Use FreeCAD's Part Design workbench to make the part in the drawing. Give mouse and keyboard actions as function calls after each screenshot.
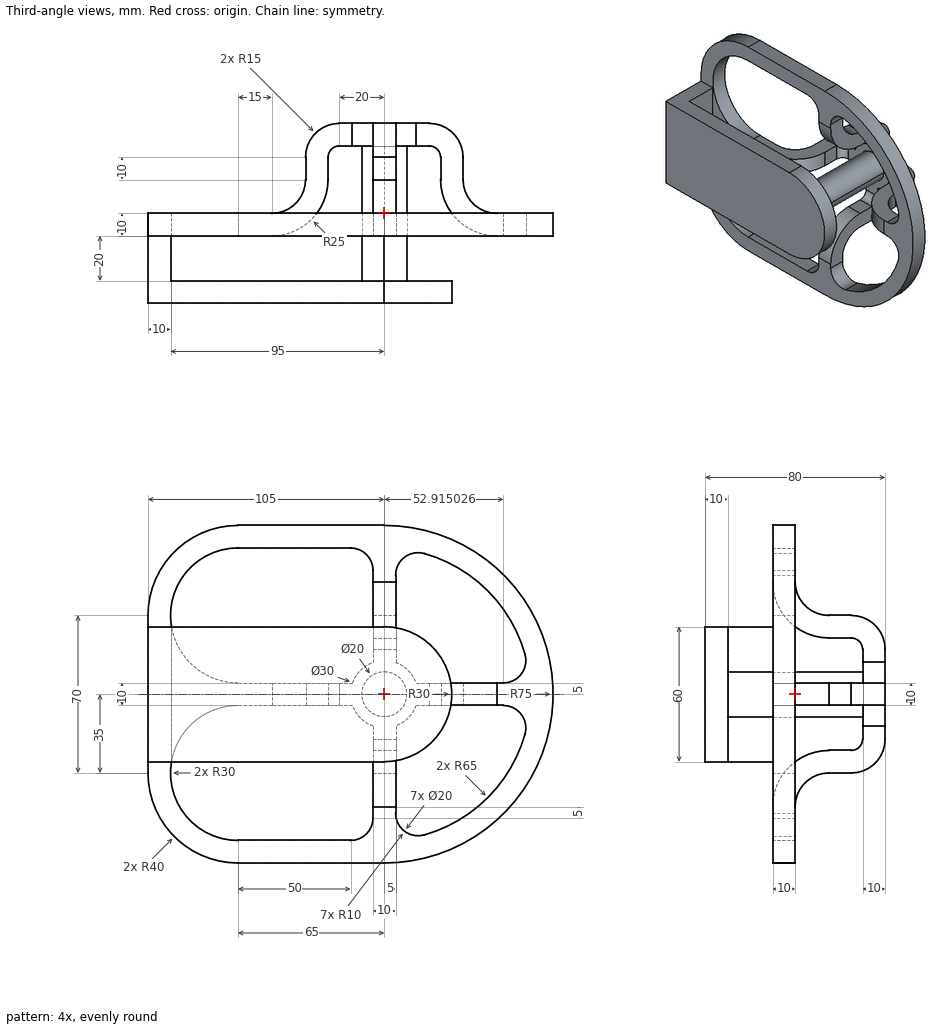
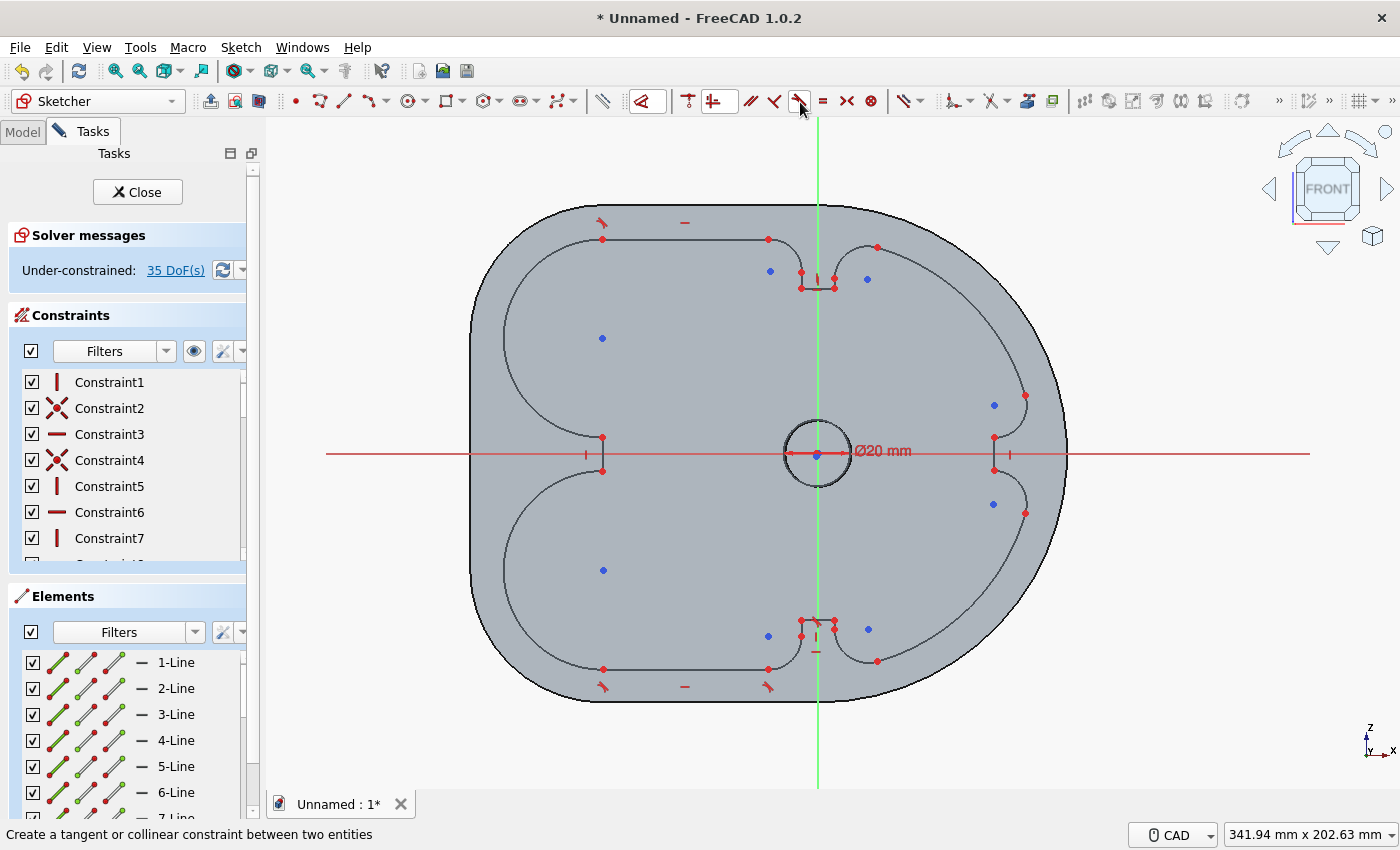
click(653, 240)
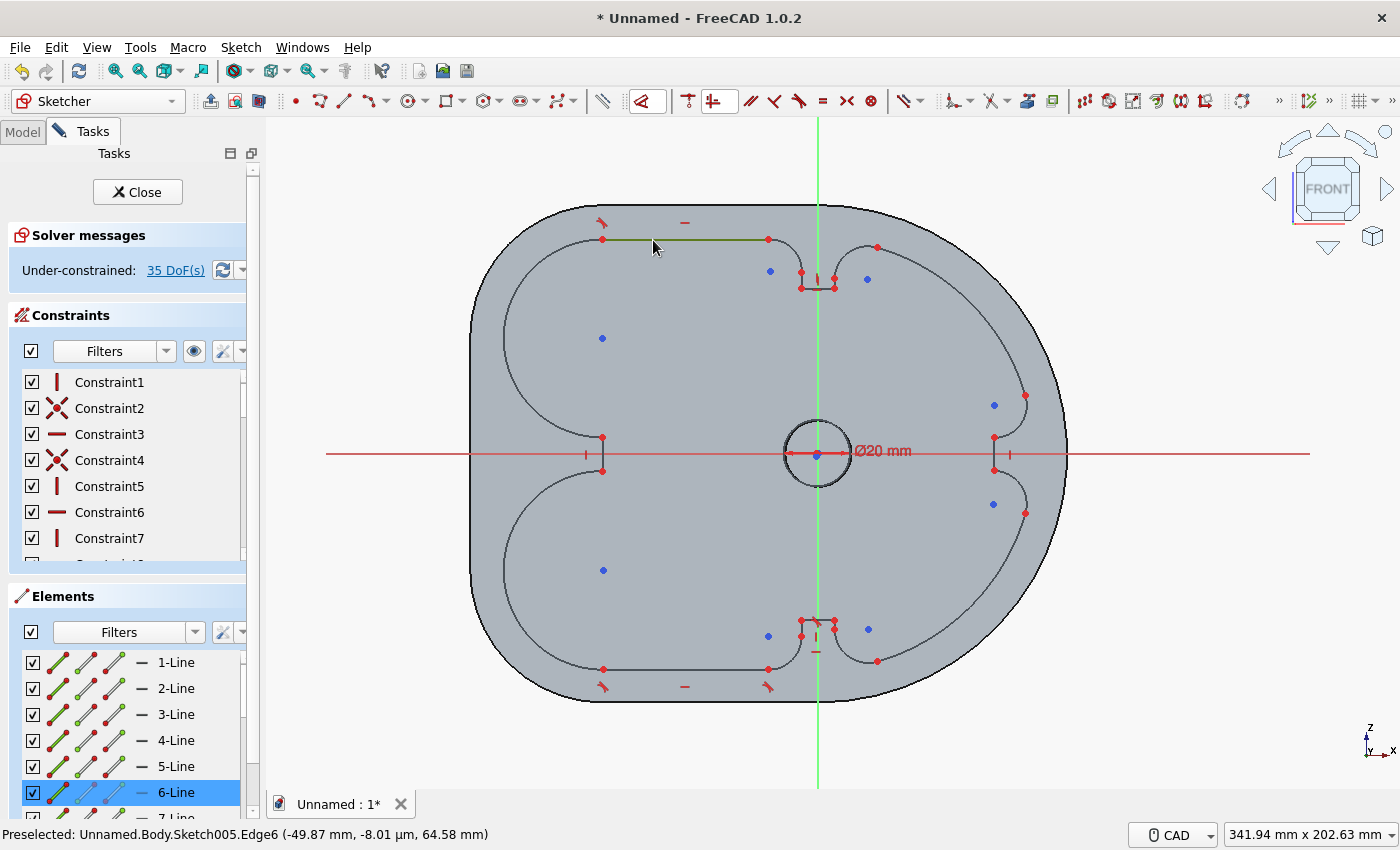
click(799, 257)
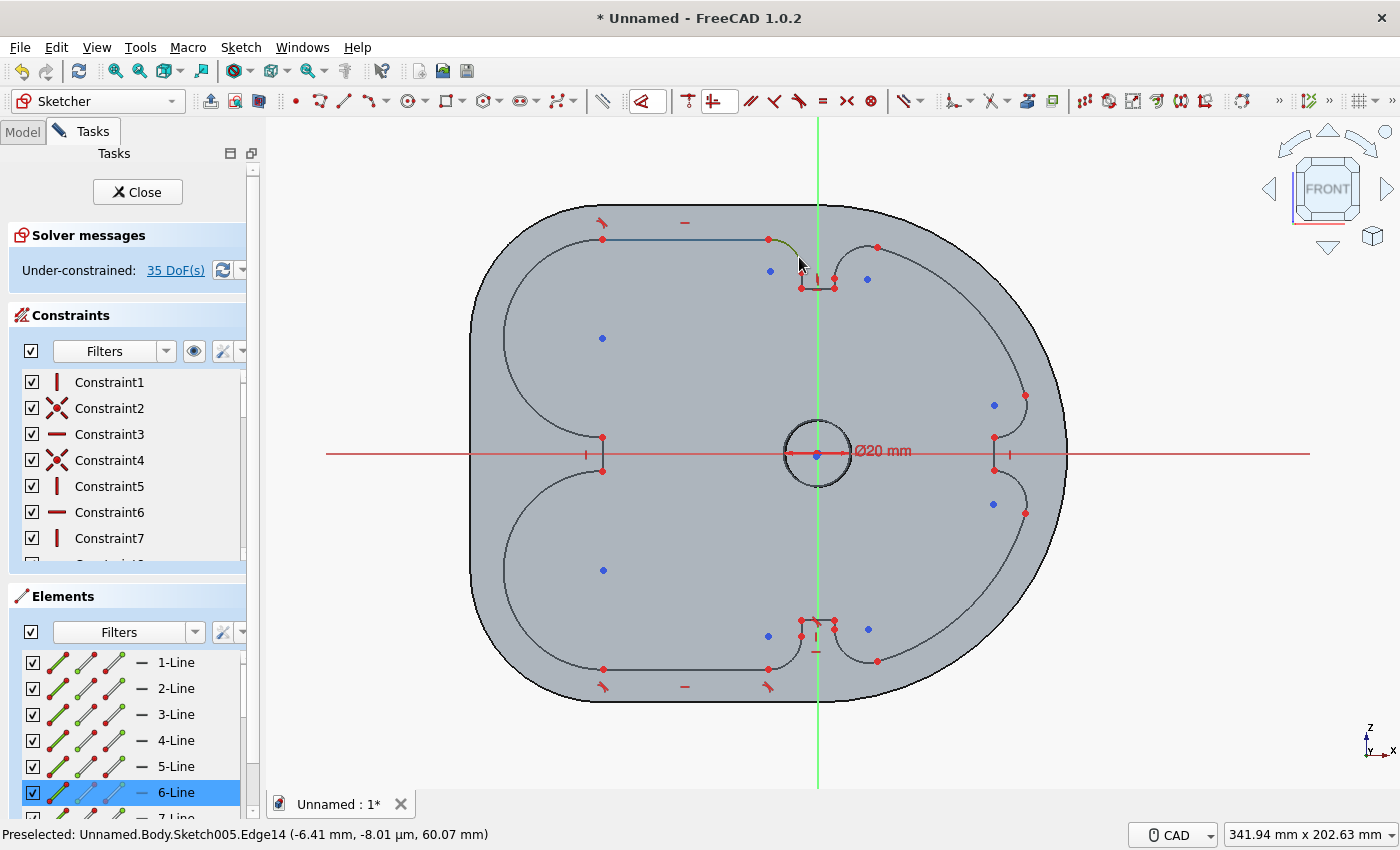
click(800, 102)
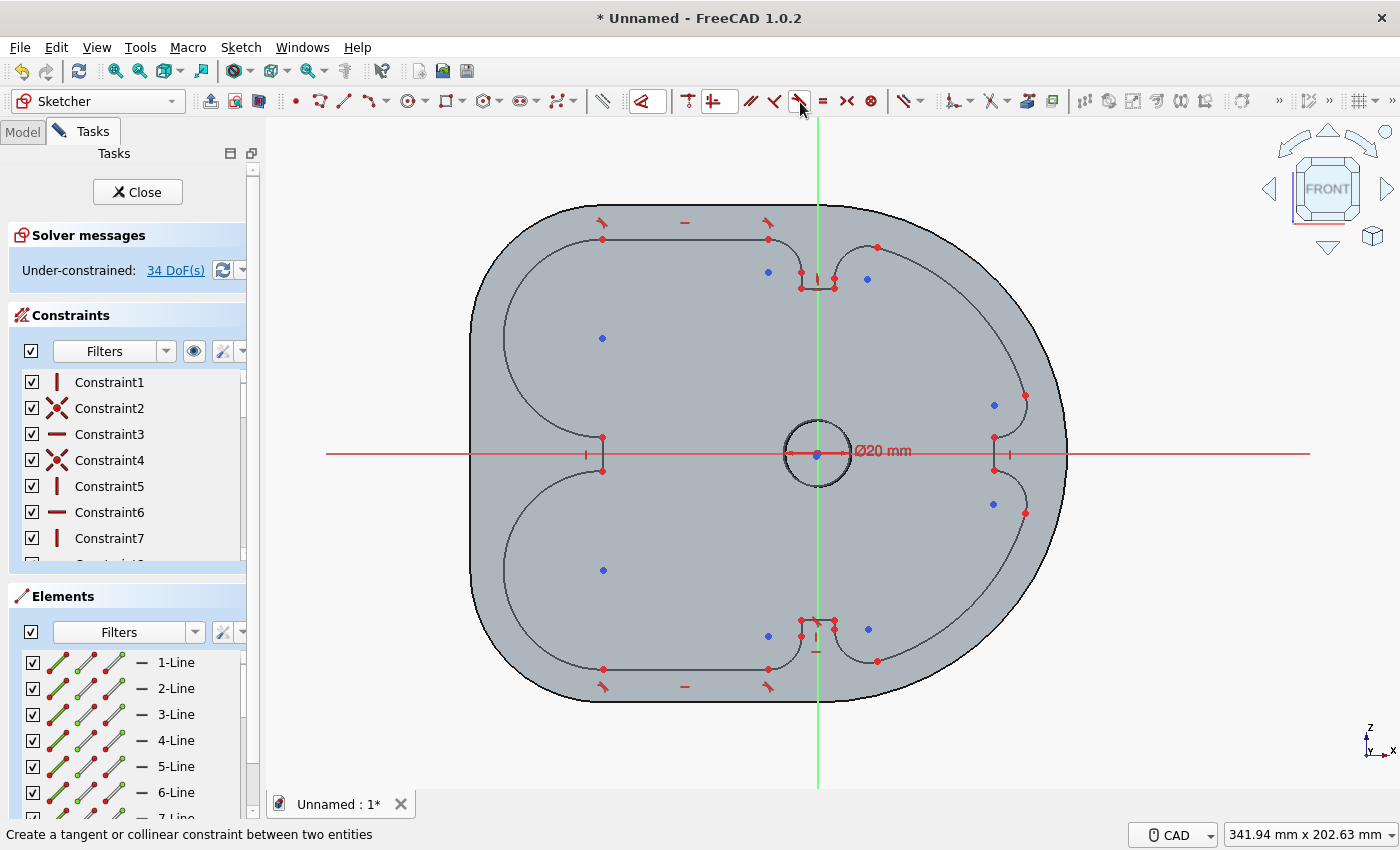
scroll(802, 281, up, 3)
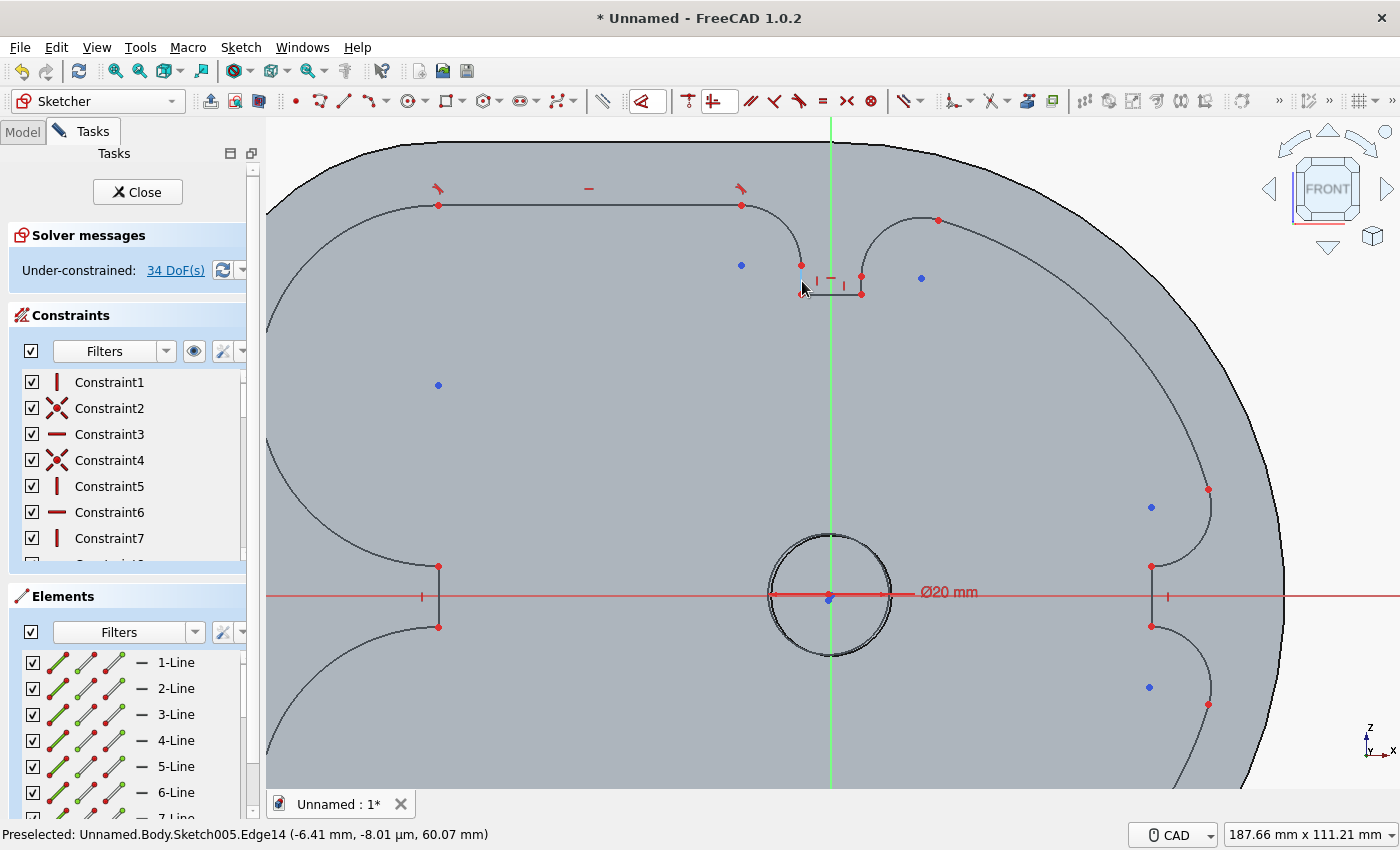
click(801, 280)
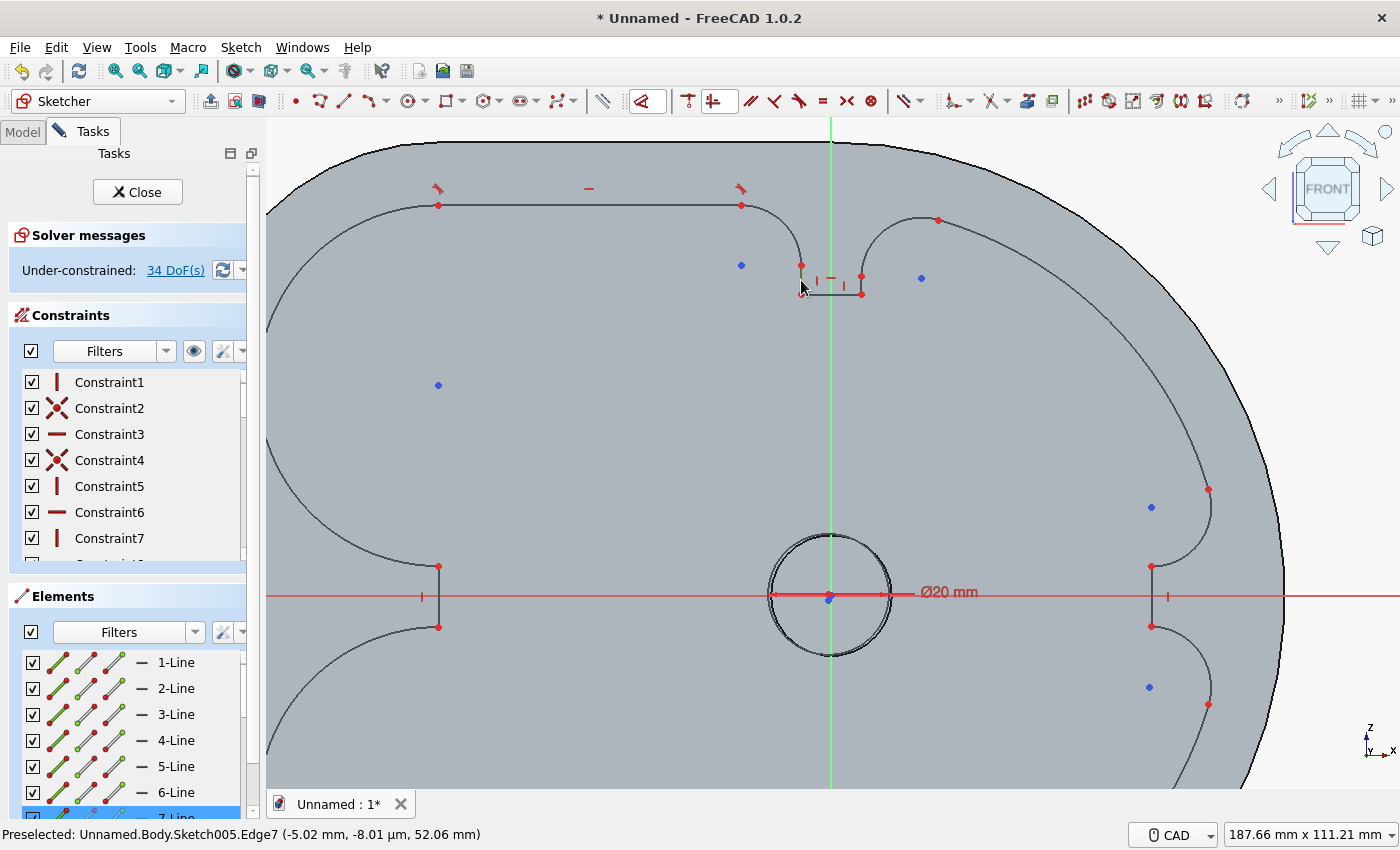
click(795, 238)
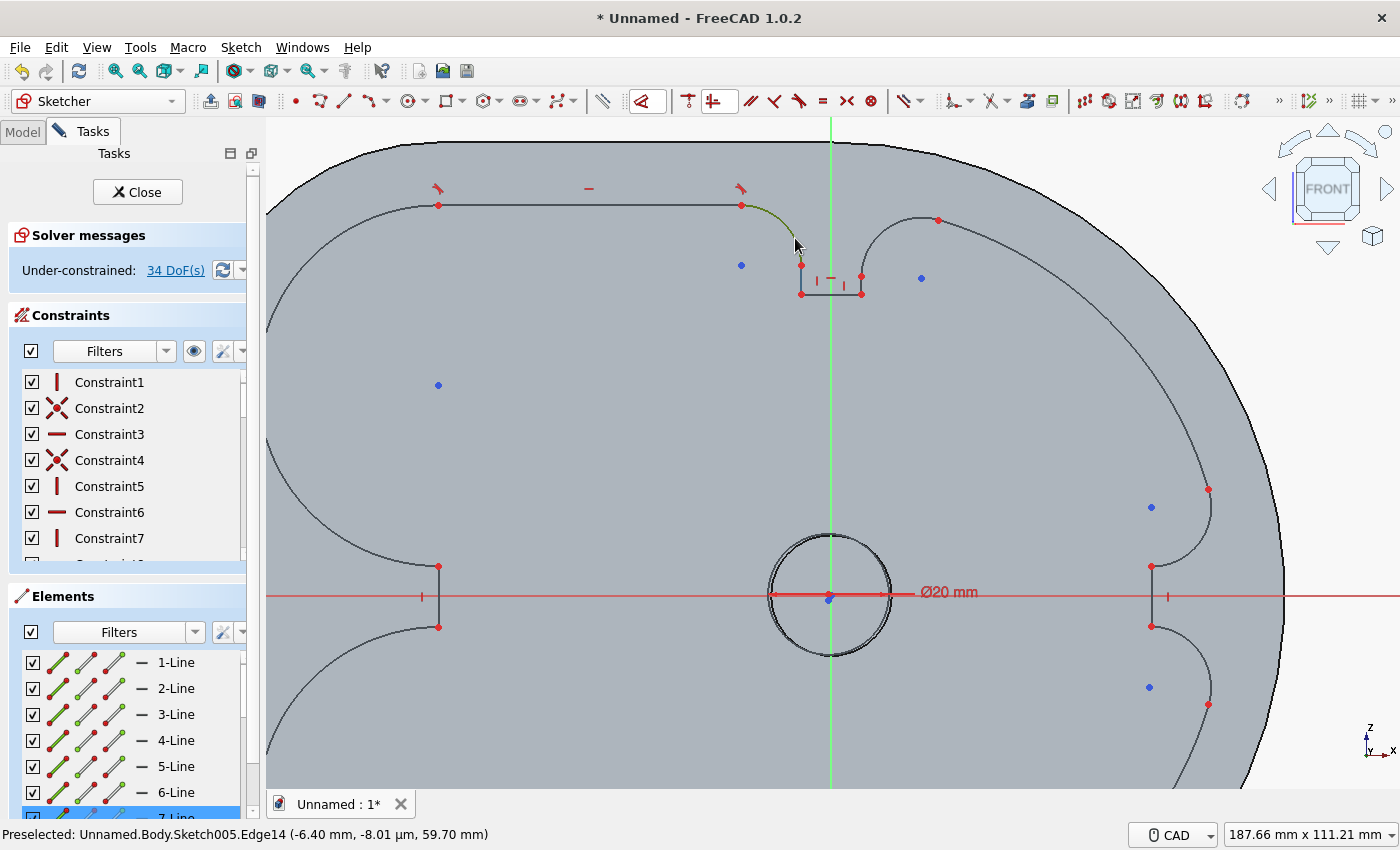
click(800, 102)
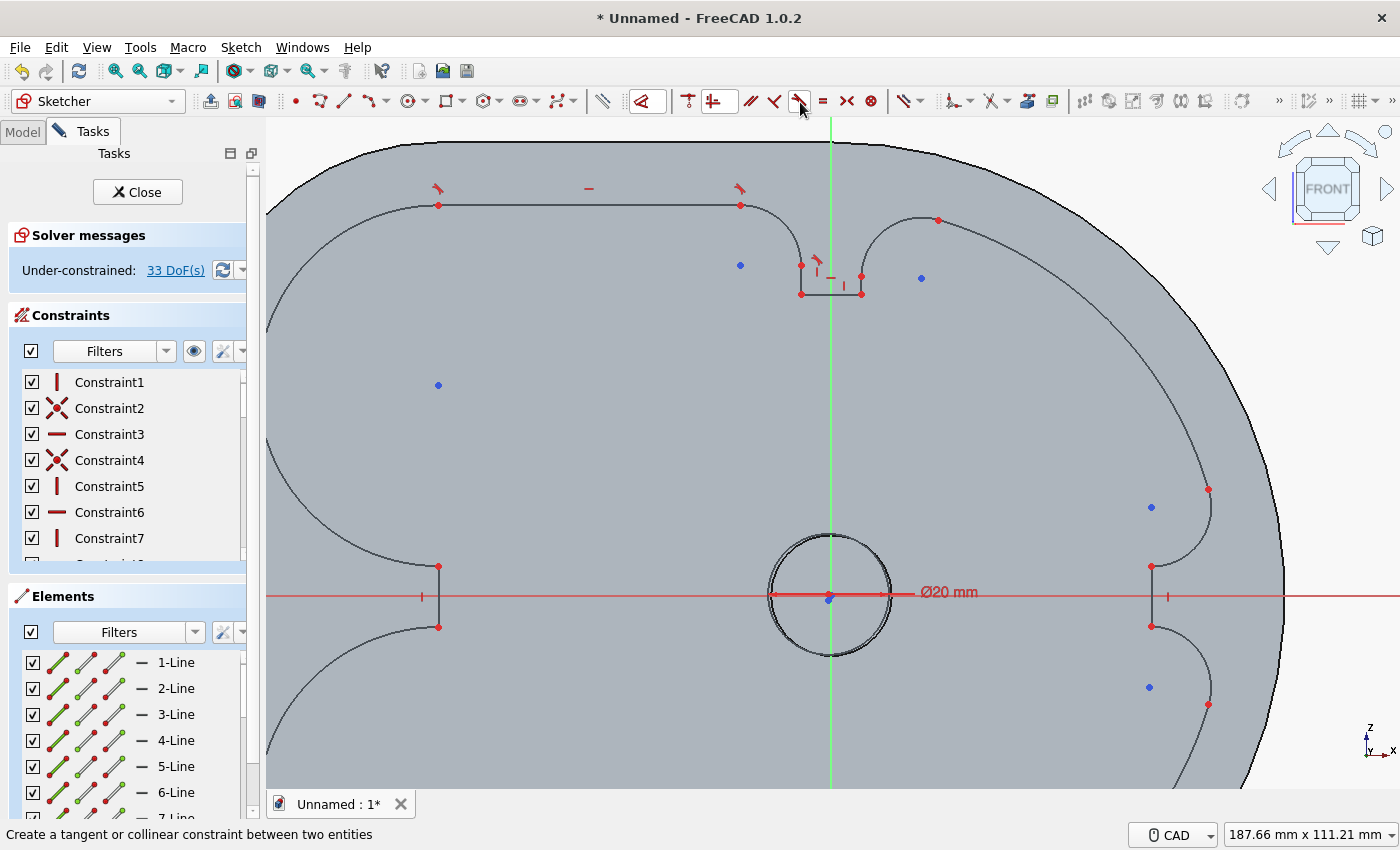
scroll(861, 286, up, 3)